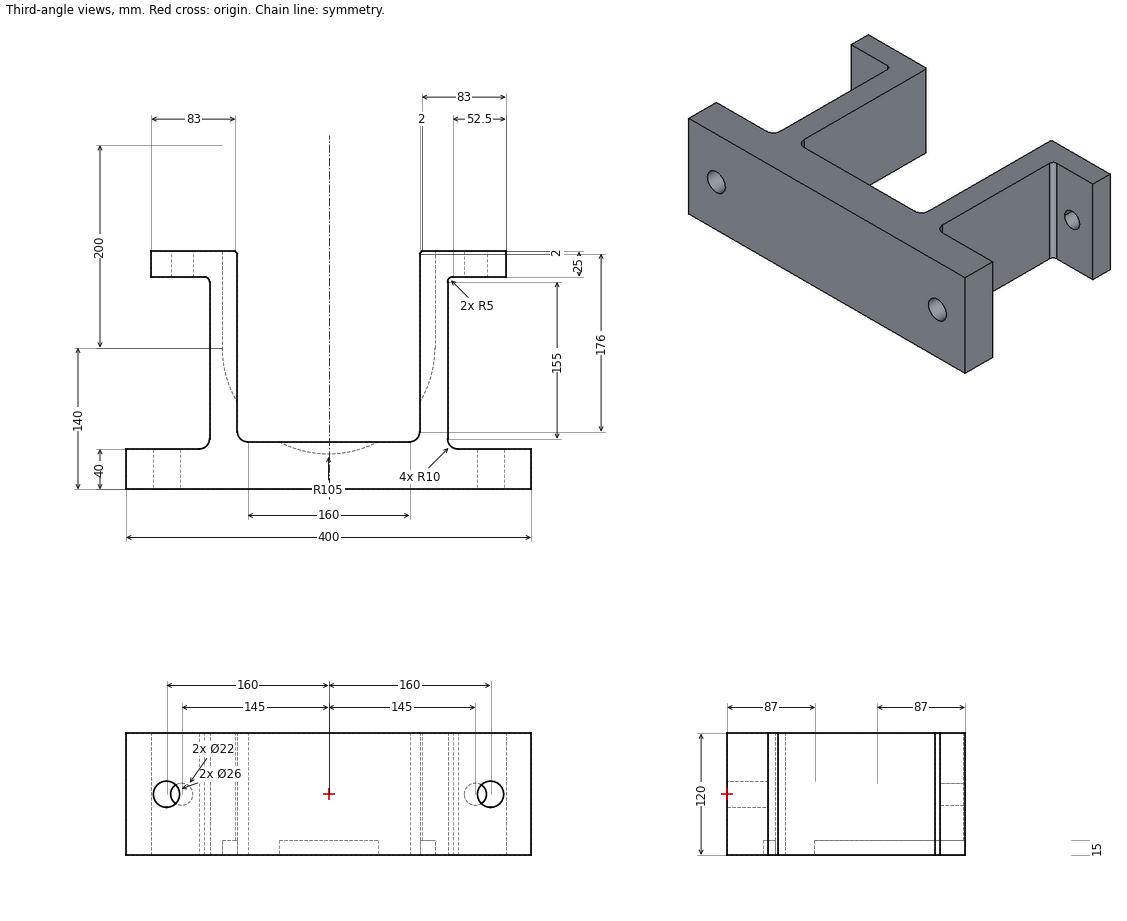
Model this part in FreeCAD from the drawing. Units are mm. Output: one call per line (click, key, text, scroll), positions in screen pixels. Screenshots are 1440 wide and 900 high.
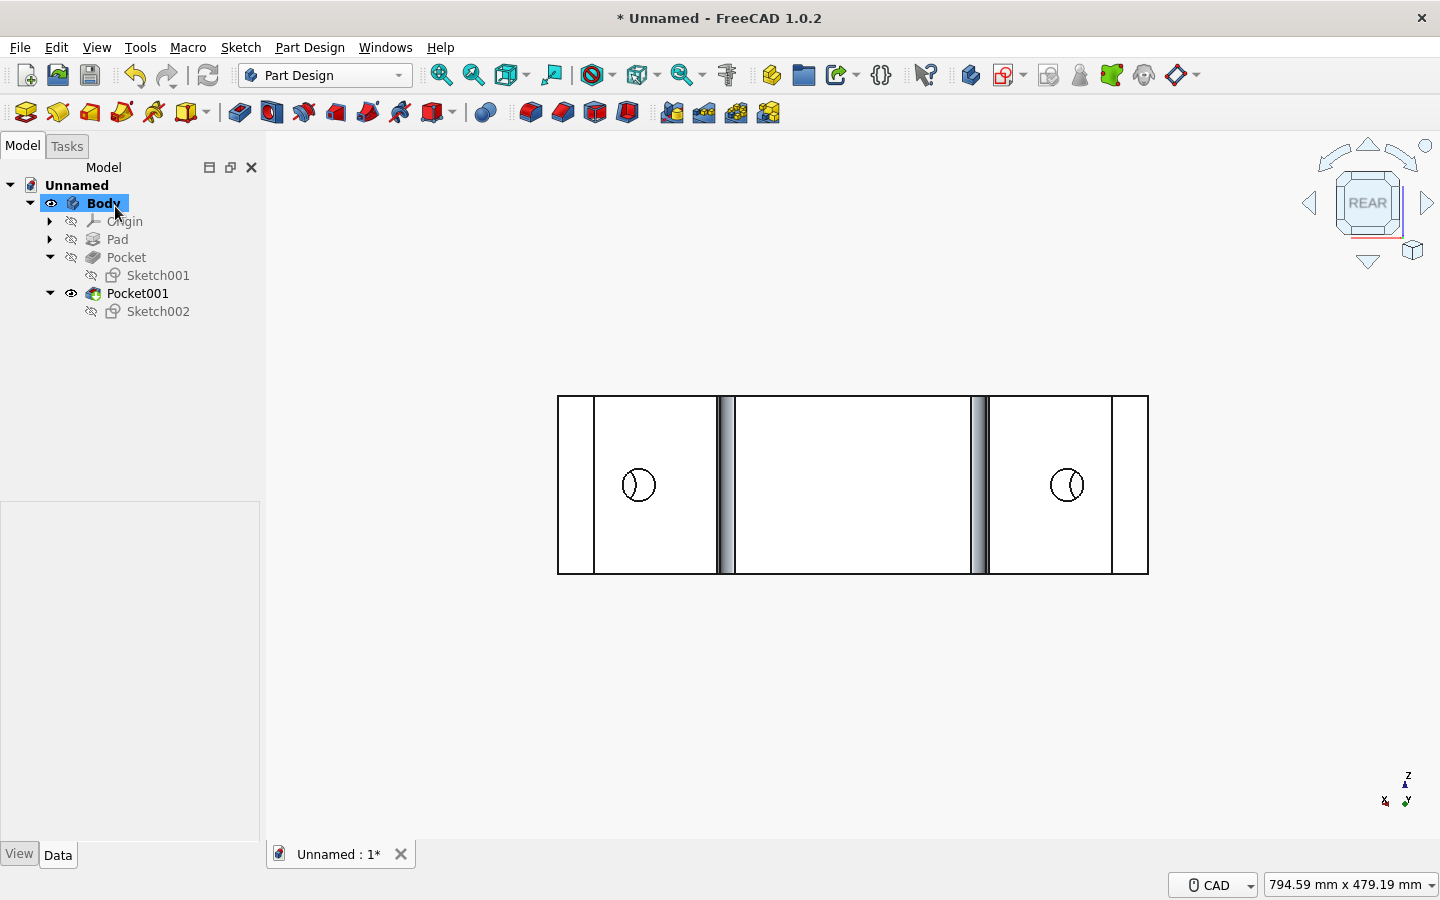
key(5)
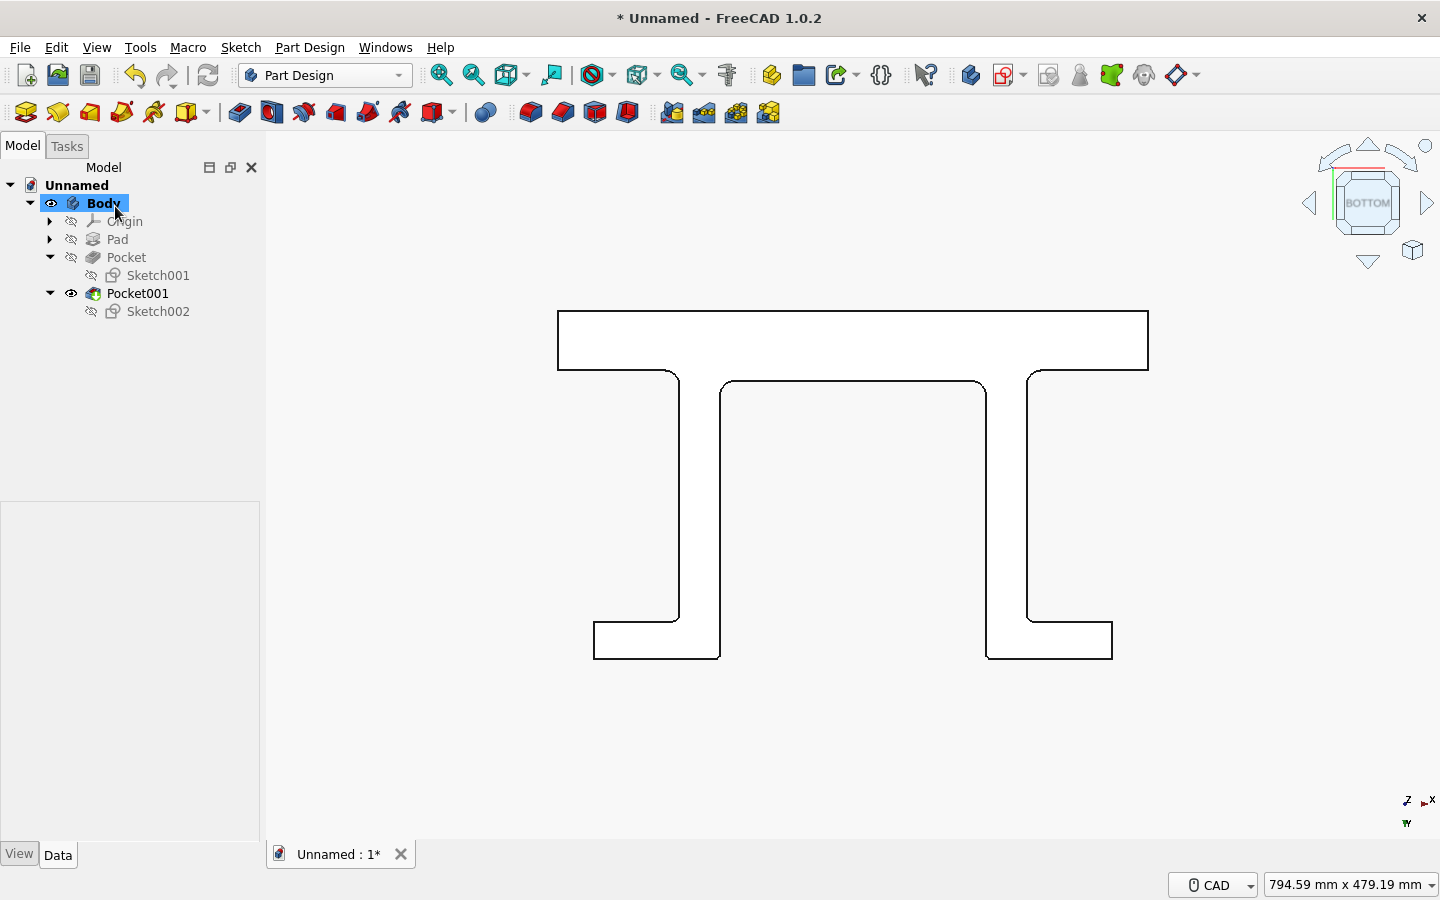
click(1106, 335)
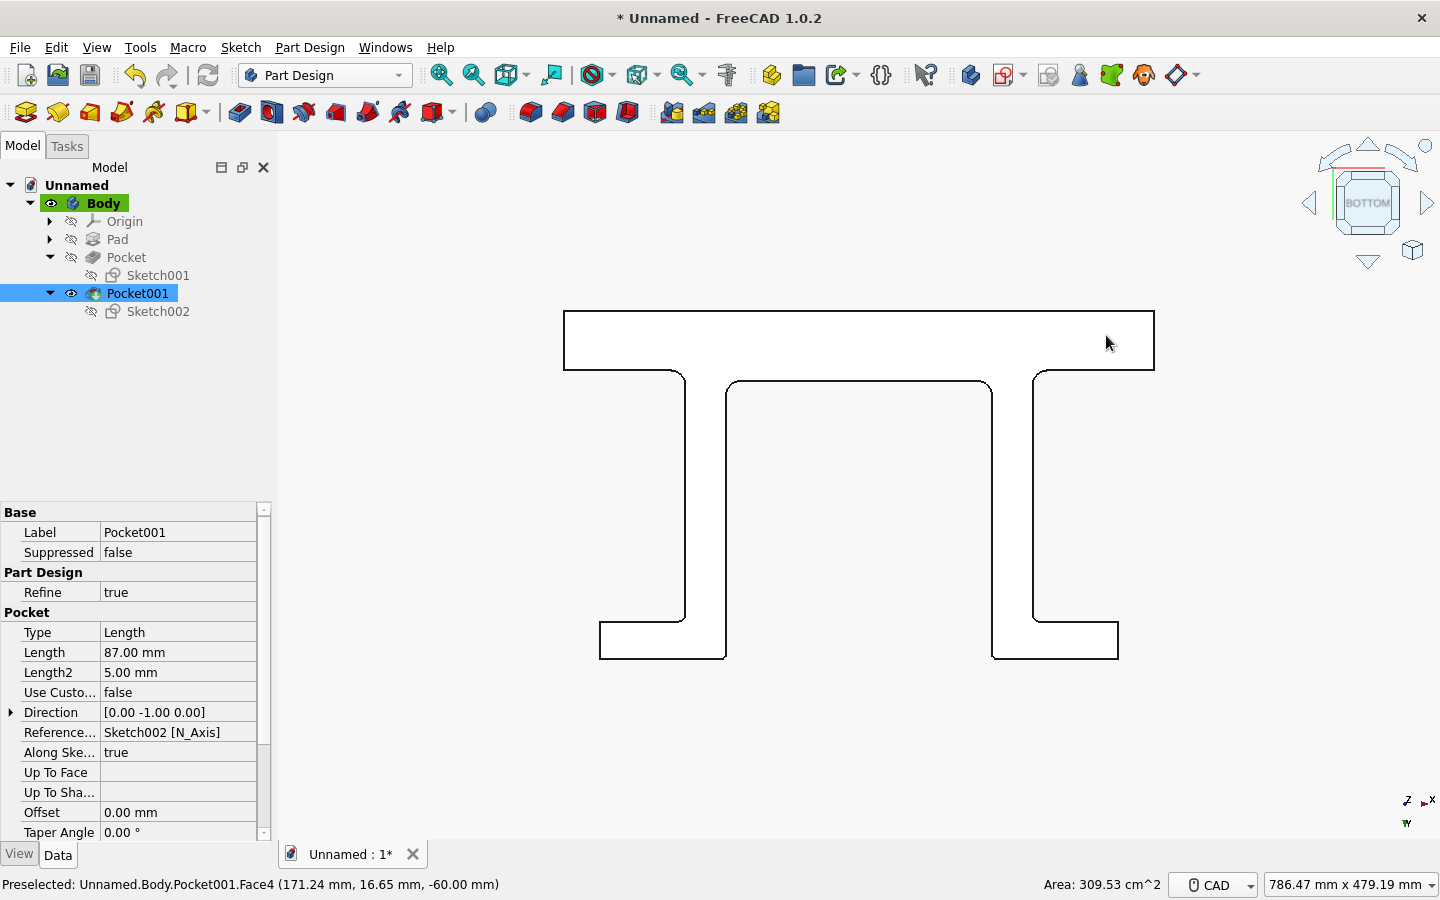
click(1004, 76)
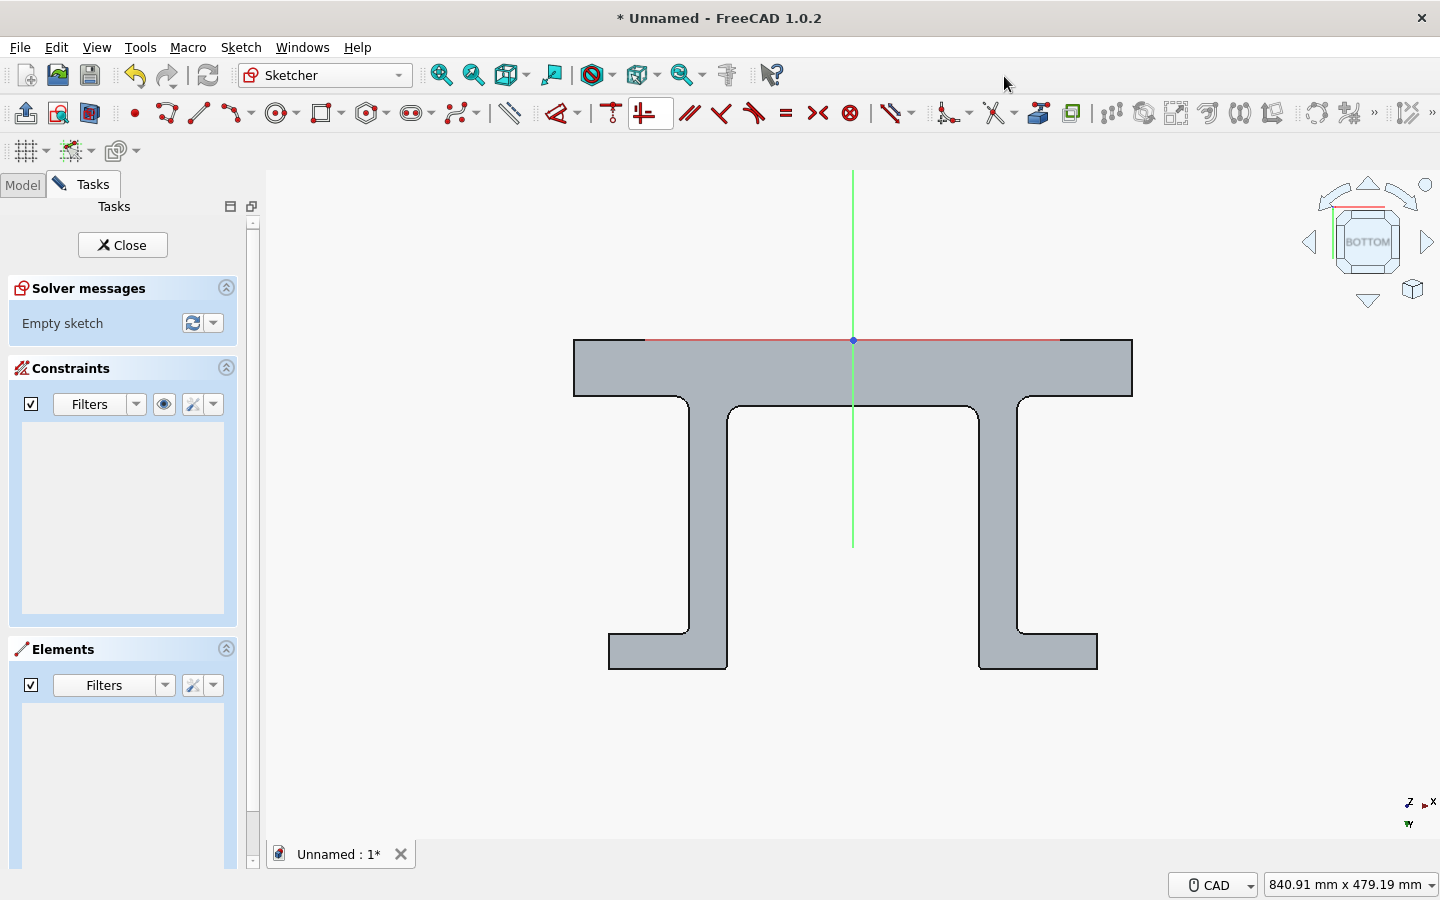
scroll(475, 198, down, 1)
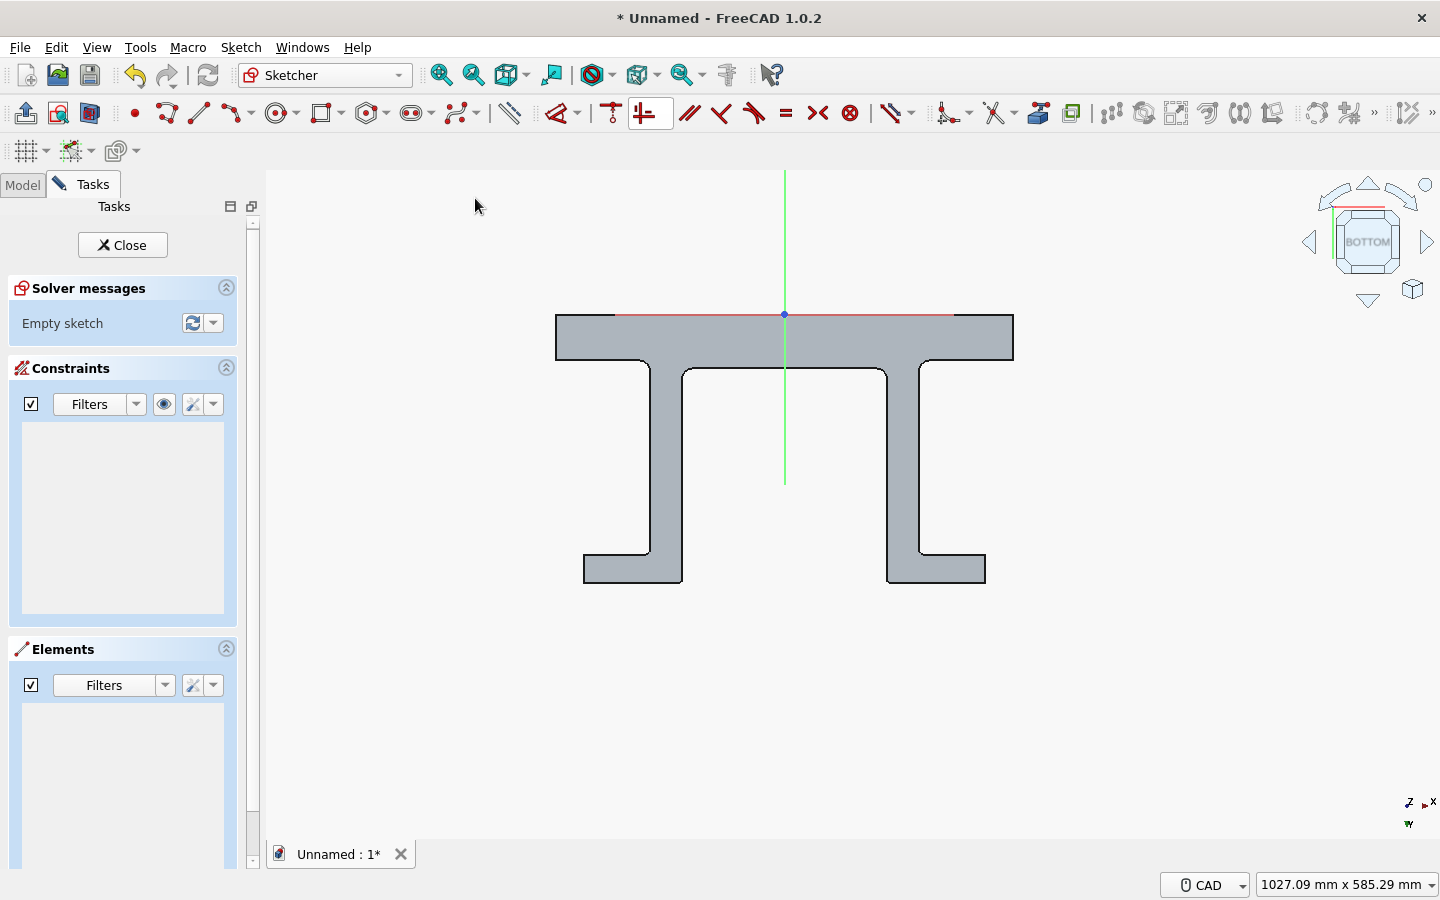
click(168, 114)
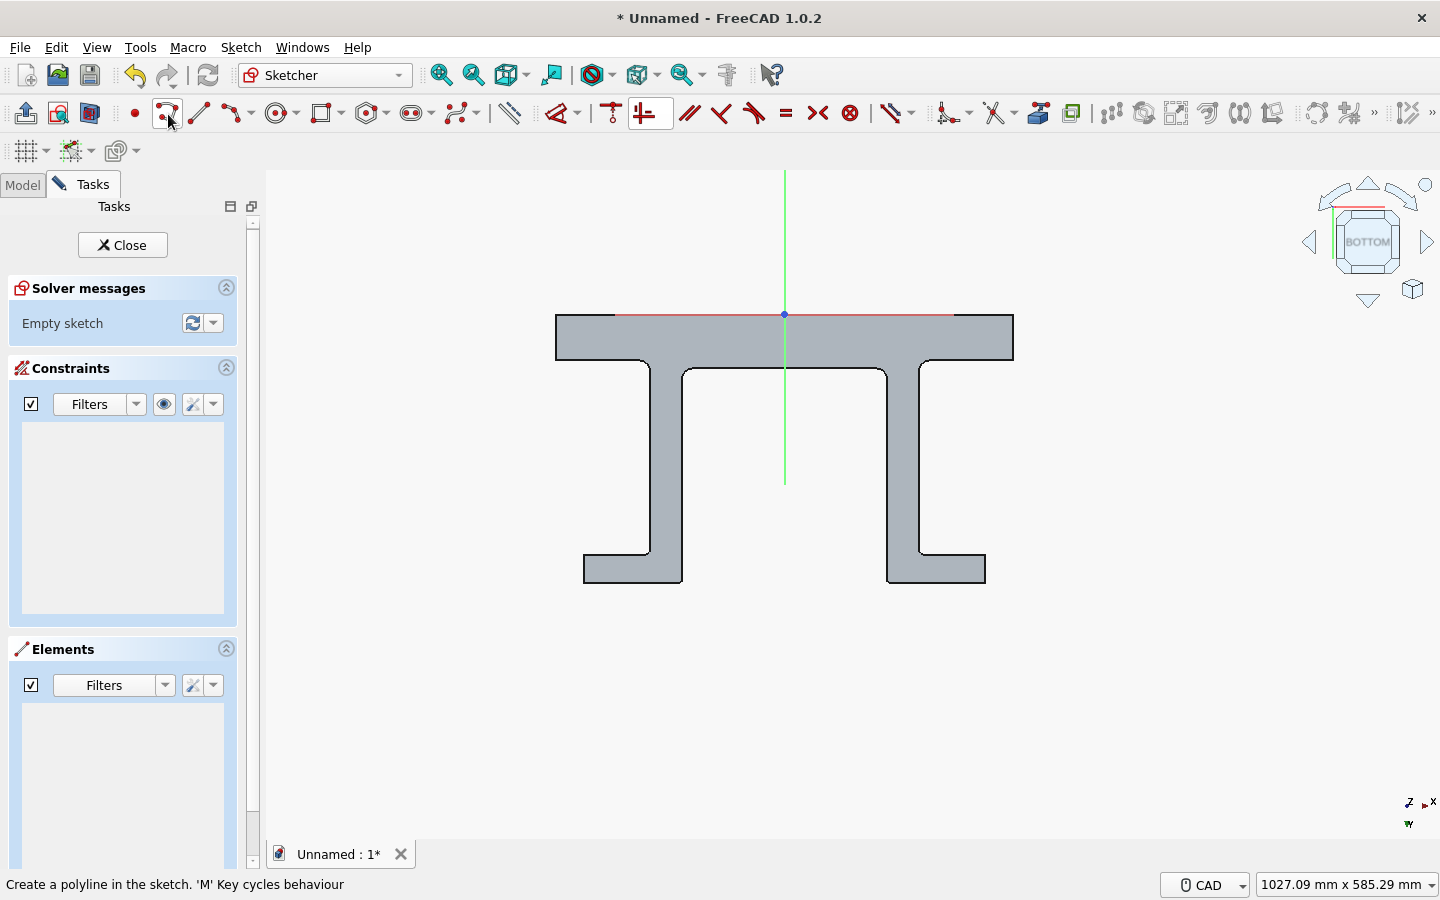
click(664, 475)
click(664, 703)
click(905, 703)
click(905, 475)
right_click(905, 475)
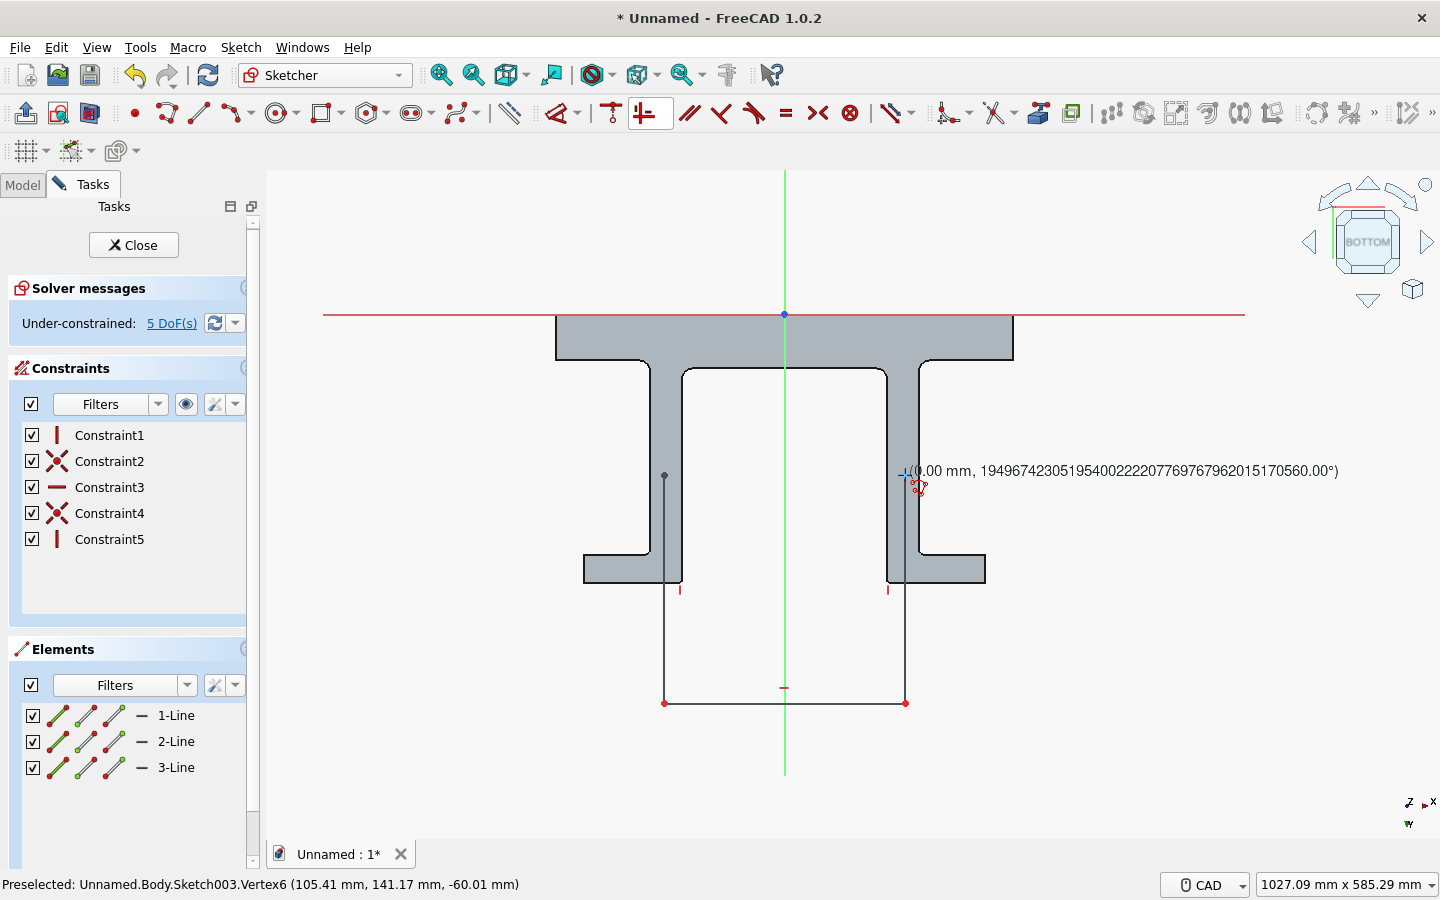
key(g)
key(3)
key(a)